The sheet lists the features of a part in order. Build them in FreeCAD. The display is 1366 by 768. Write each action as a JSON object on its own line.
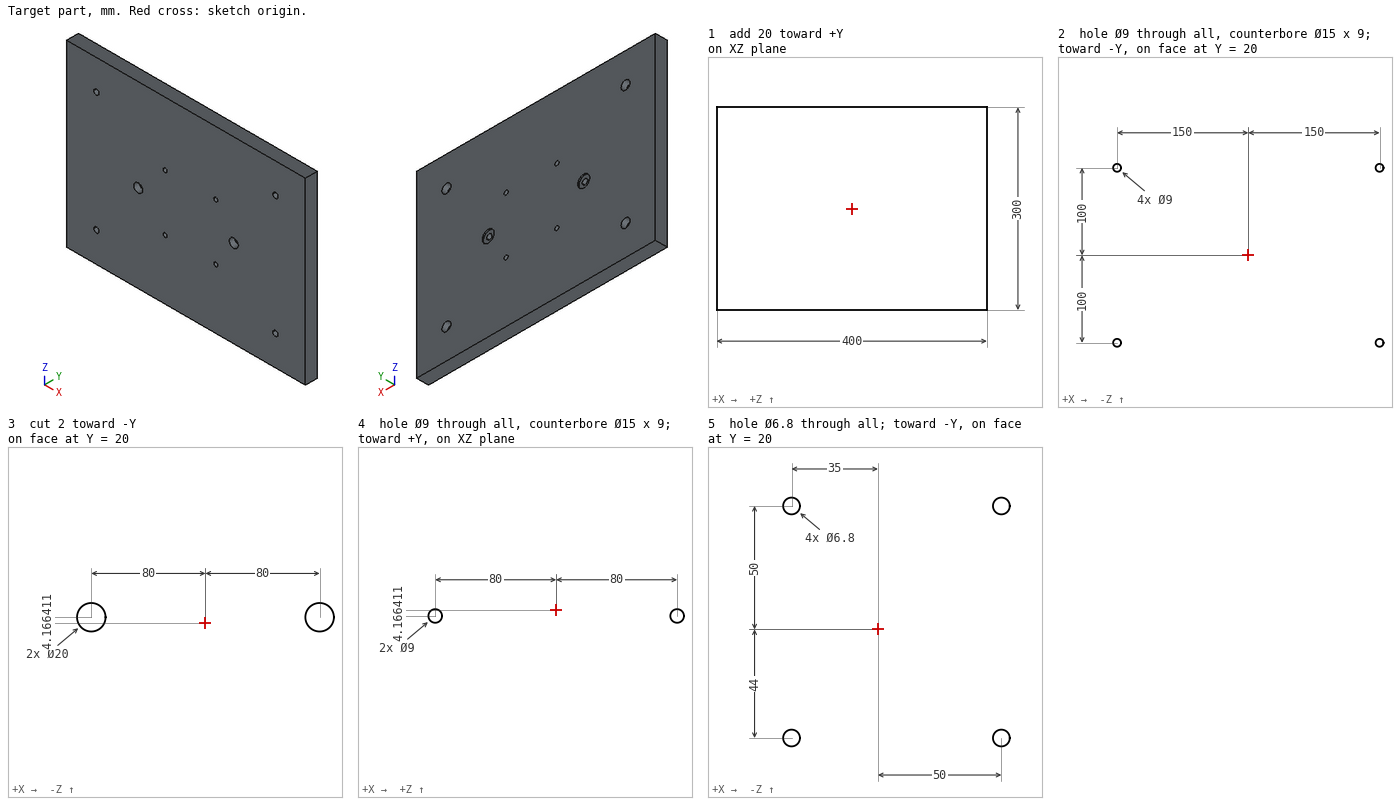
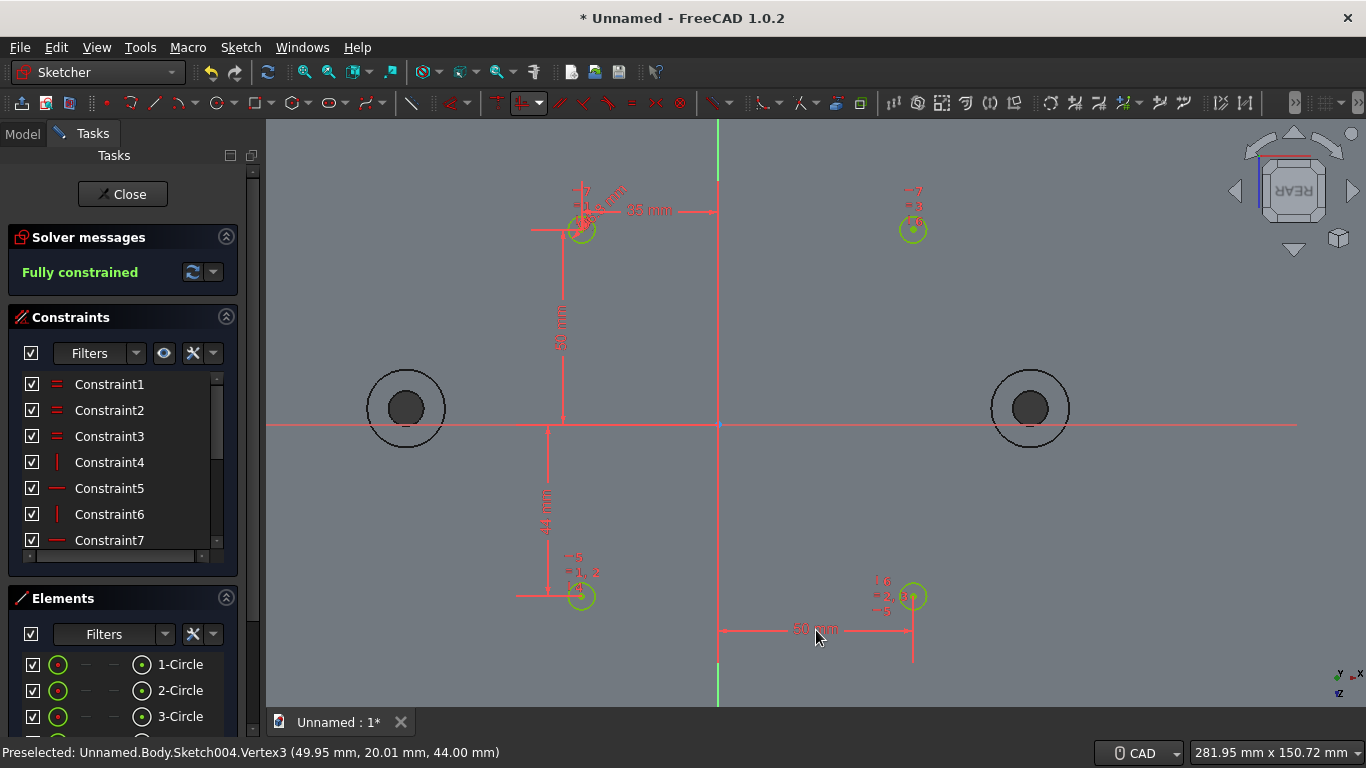
{"action": "left_click", "coordinate": [123, 194]}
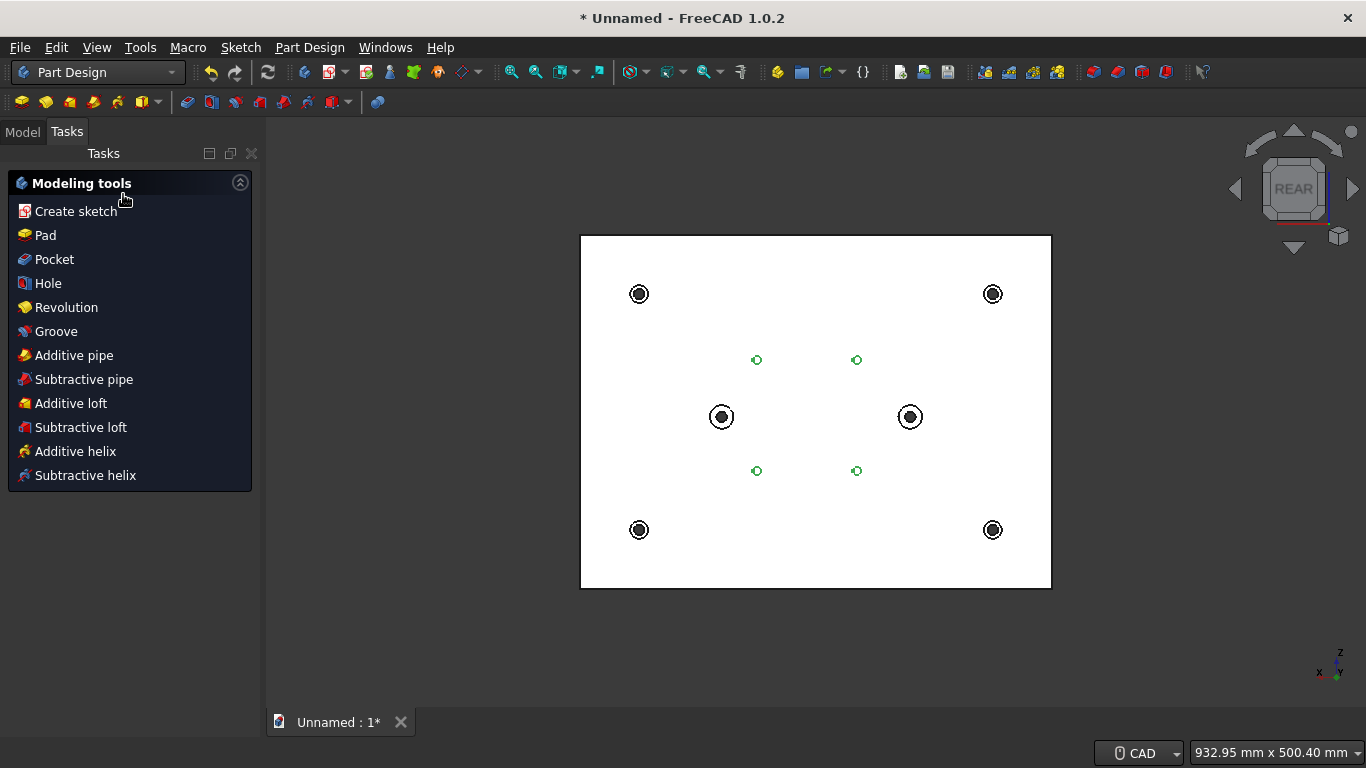
{"action": "left_click", "coordinate": [212, 102]}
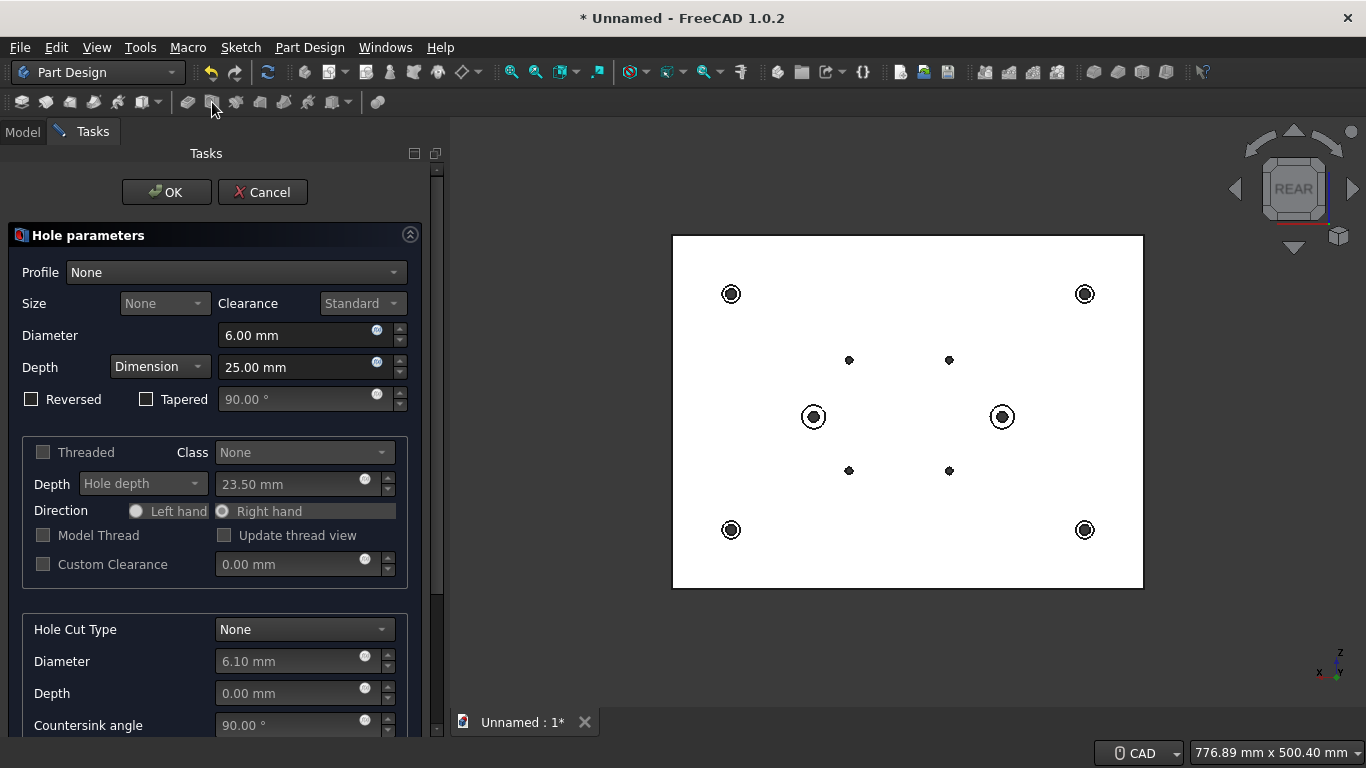
{"action": "triple_click", "coordinate": [305, 335]}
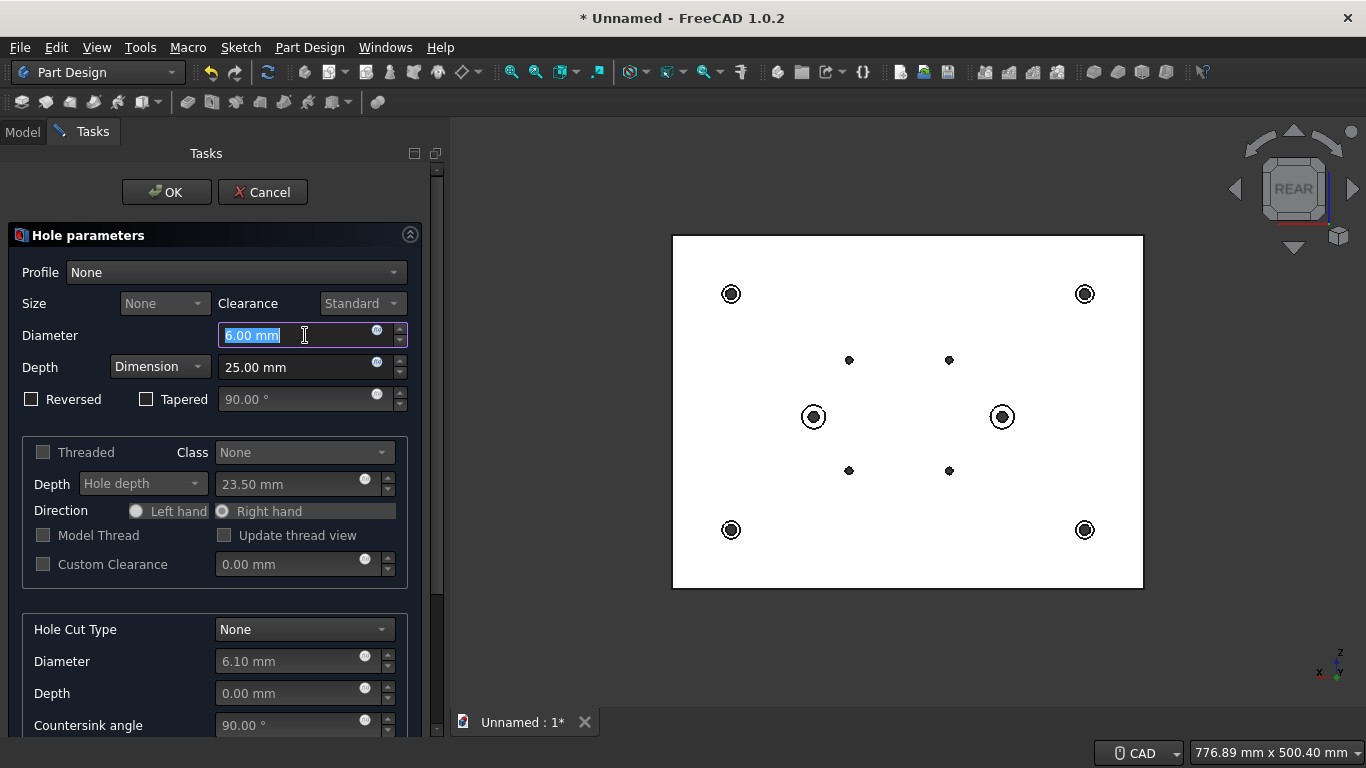
{"action": "type", "text": "6.8"}
{"action": "key", "text": "Tab"}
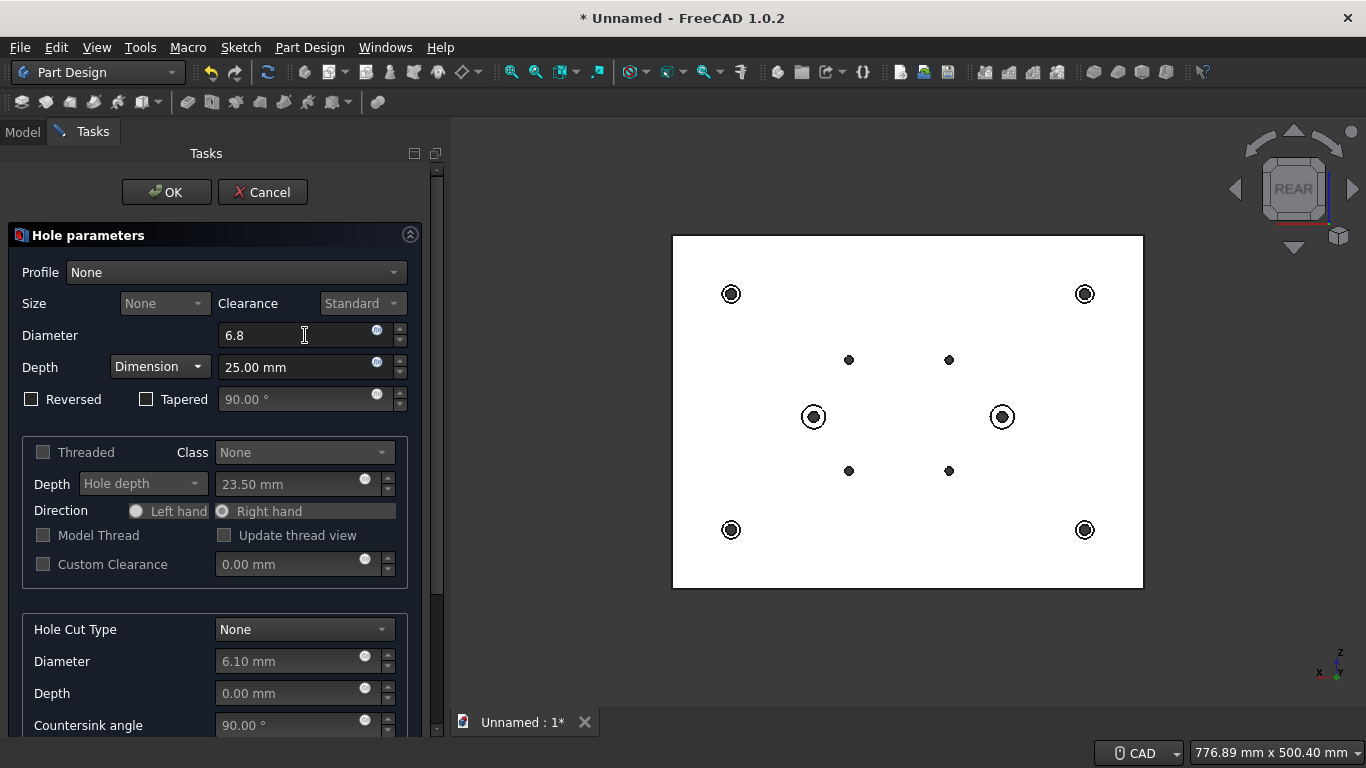
{"action": "left_click", "coordinate": [161, 366]}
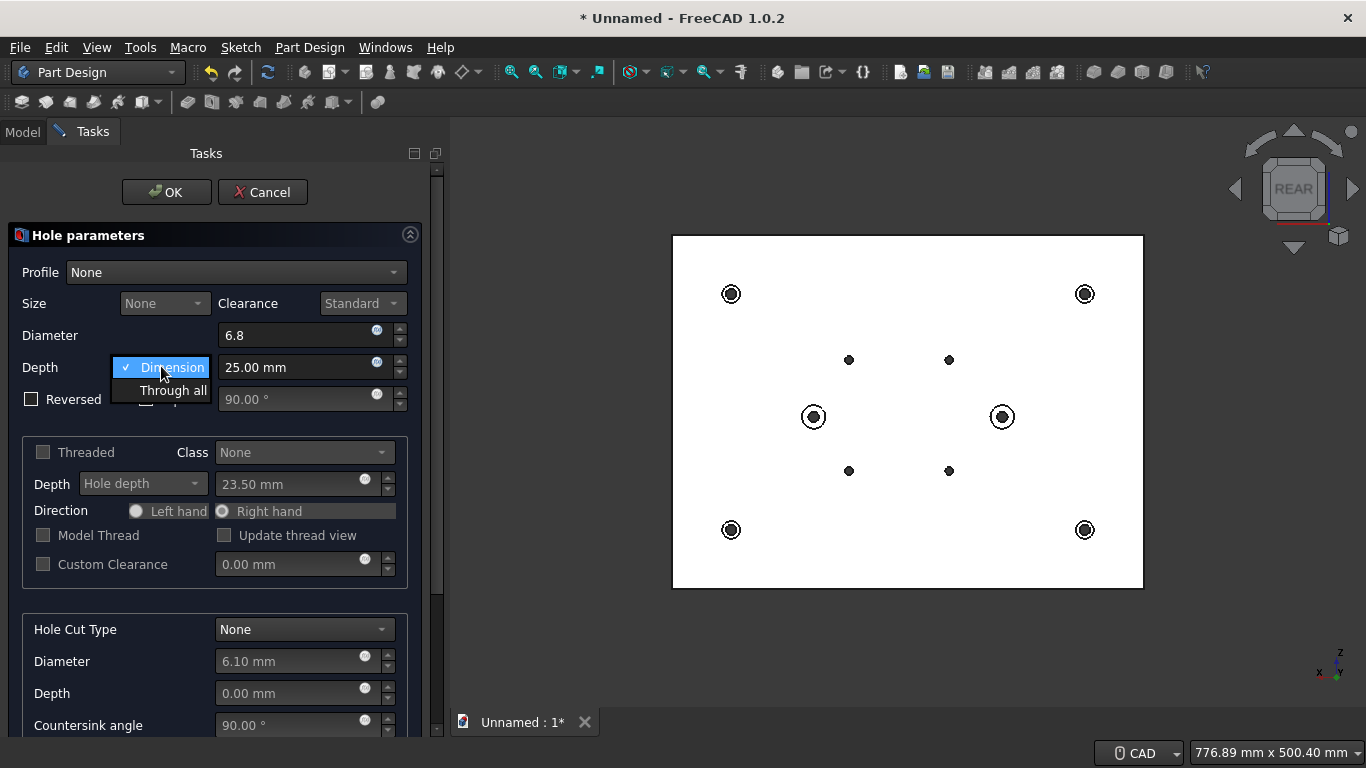
{"action": "left_click", "coordinate": [160, 390]}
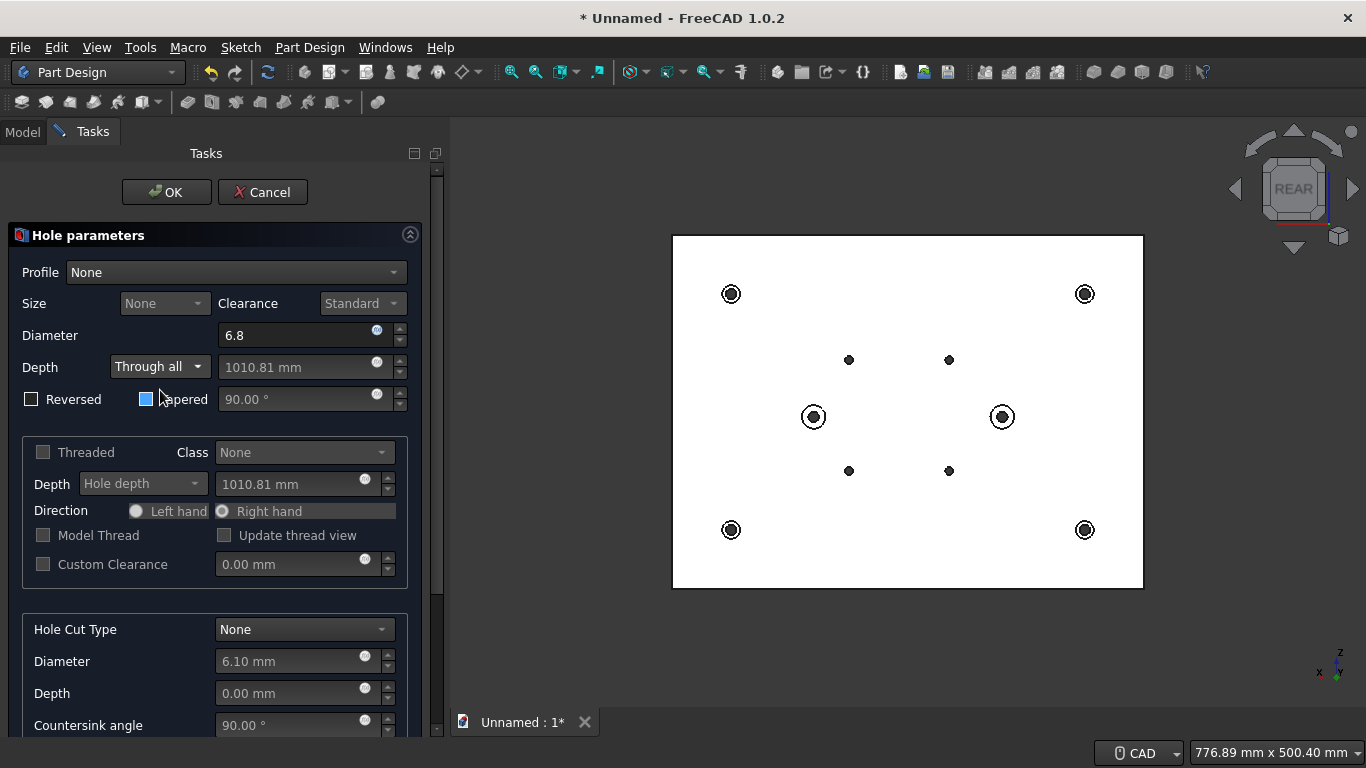
{"action": "left_click", "coordinate": [167, 192]}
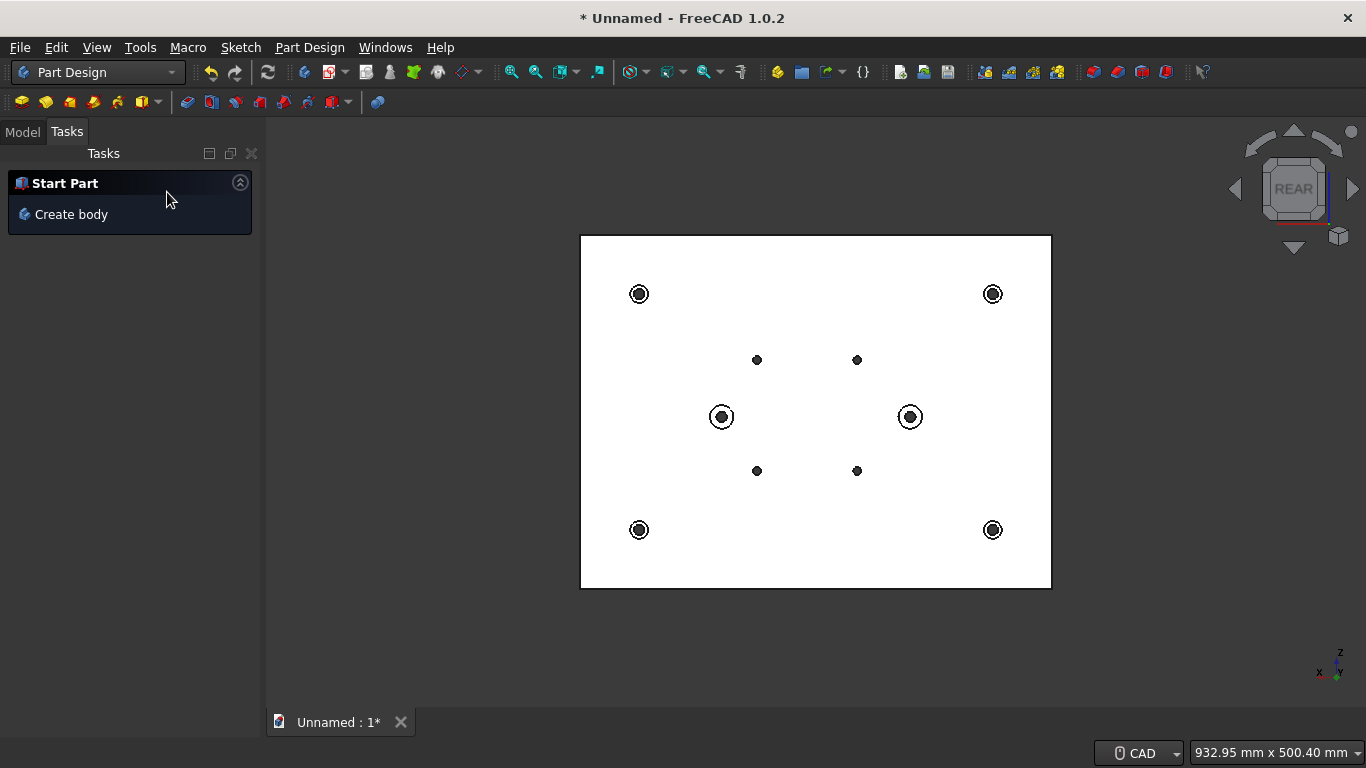
{"action": "key", "text": "0"}